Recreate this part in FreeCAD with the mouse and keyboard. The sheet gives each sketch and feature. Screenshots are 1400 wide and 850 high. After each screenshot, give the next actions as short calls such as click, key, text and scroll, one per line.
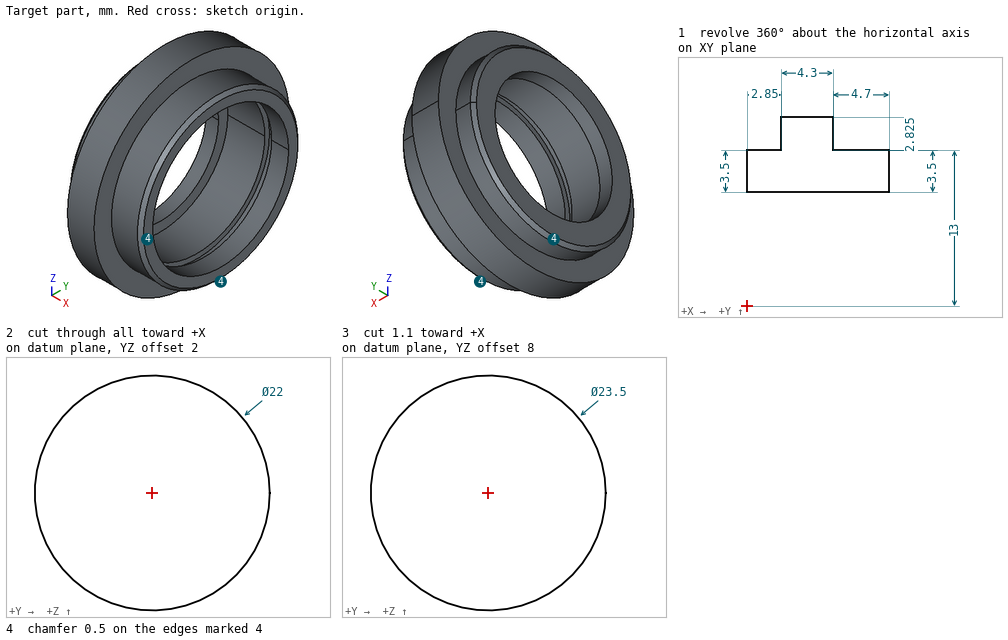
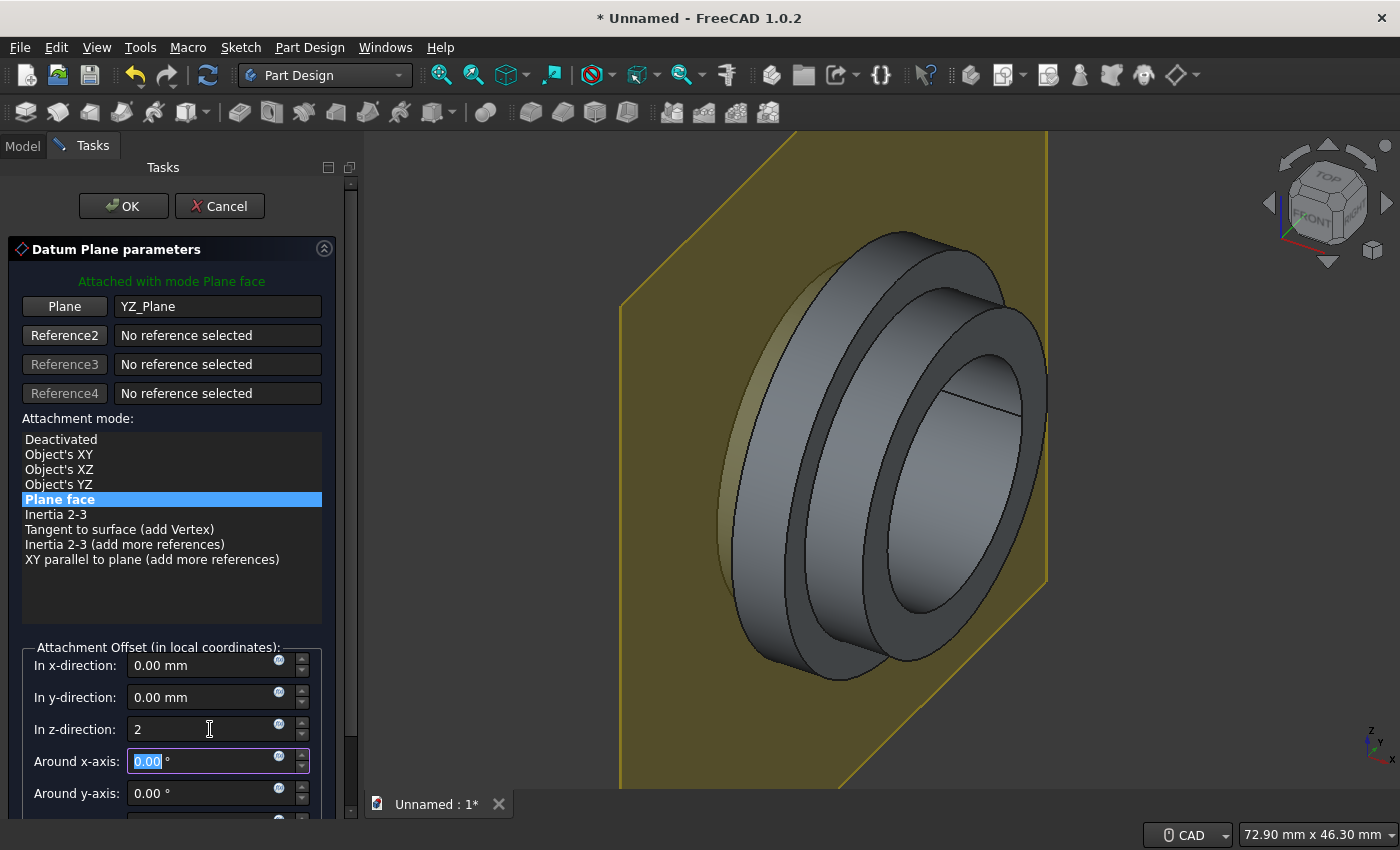
click(124, 206)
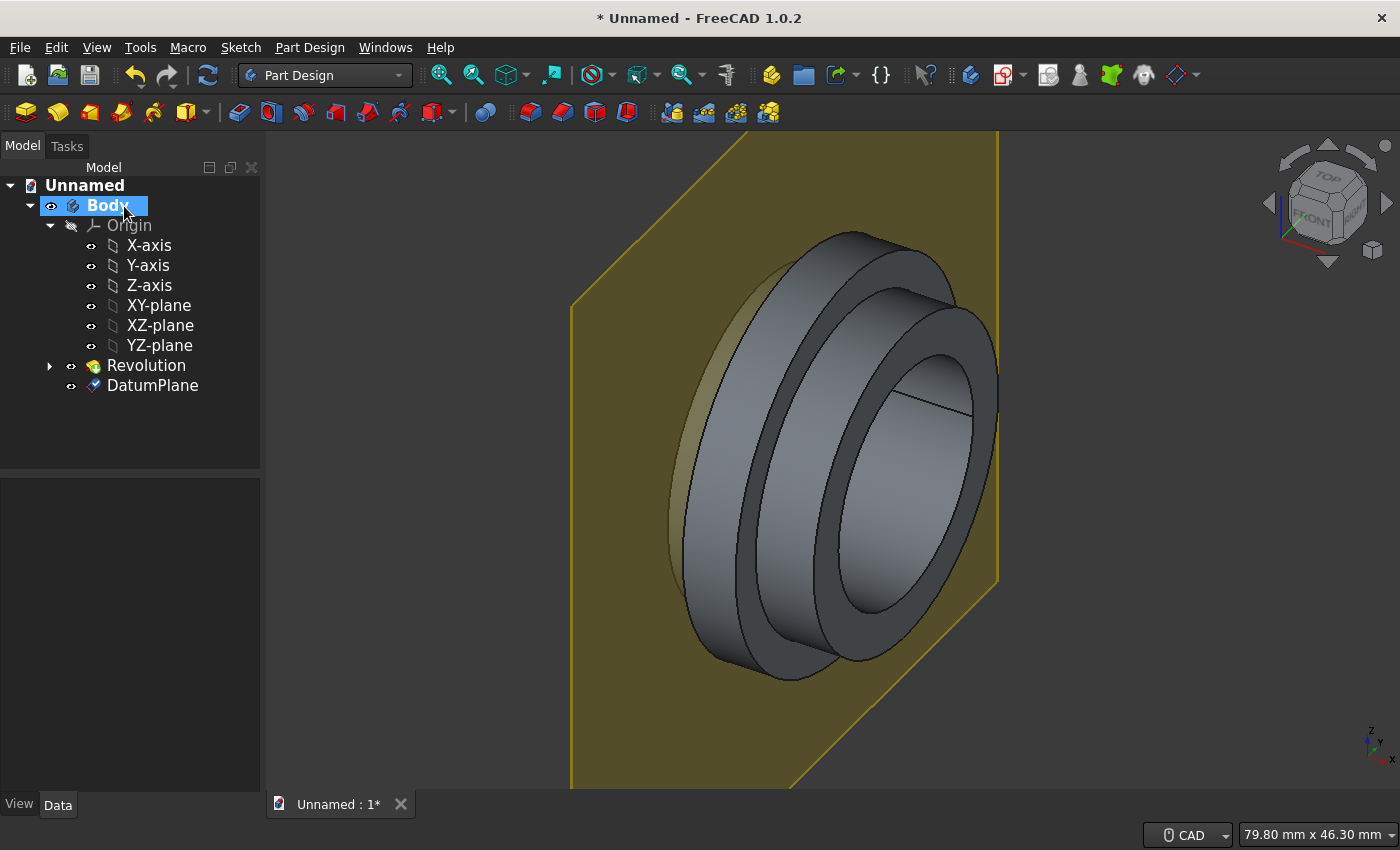
click(116, 386)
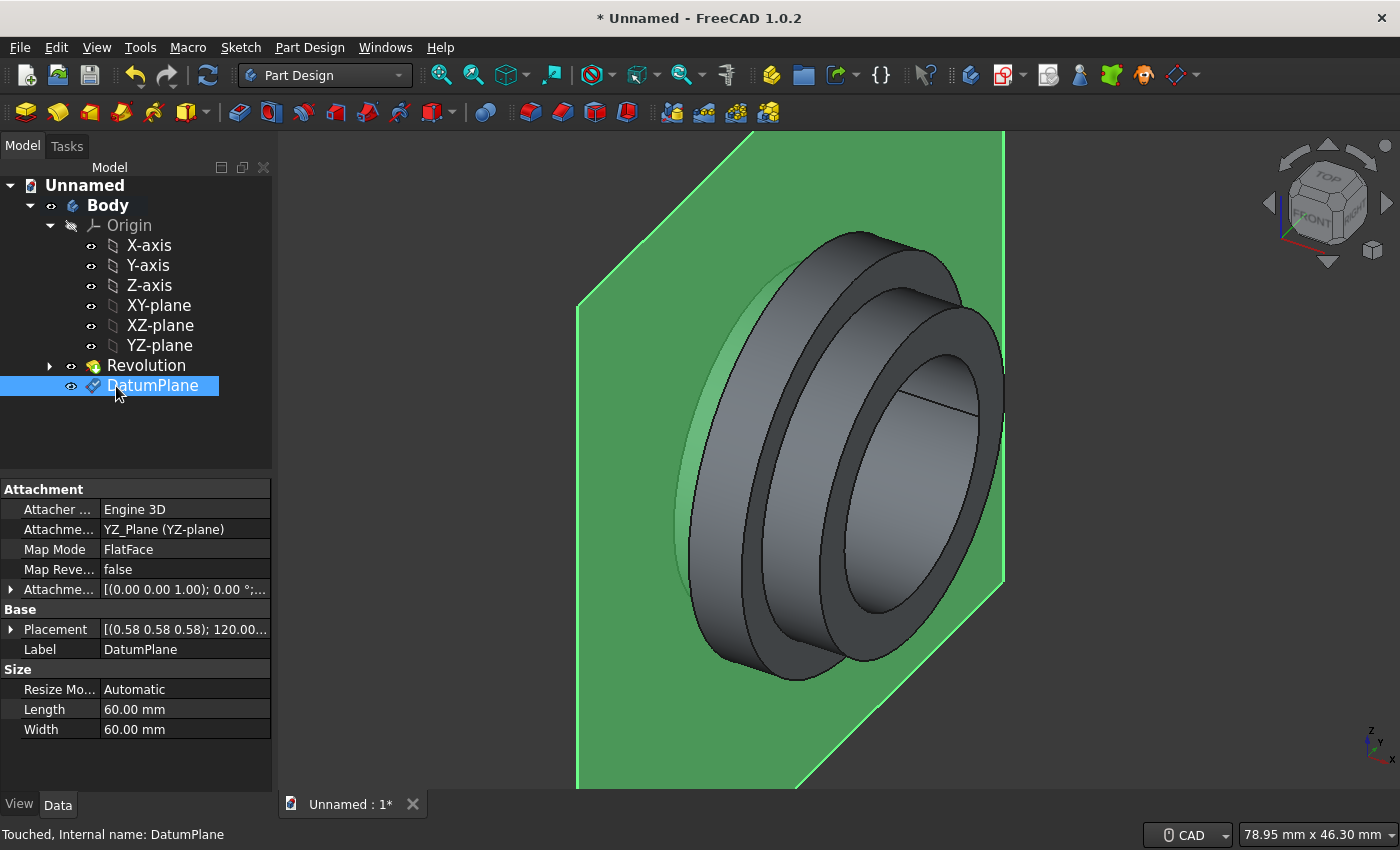
click(1004, 76)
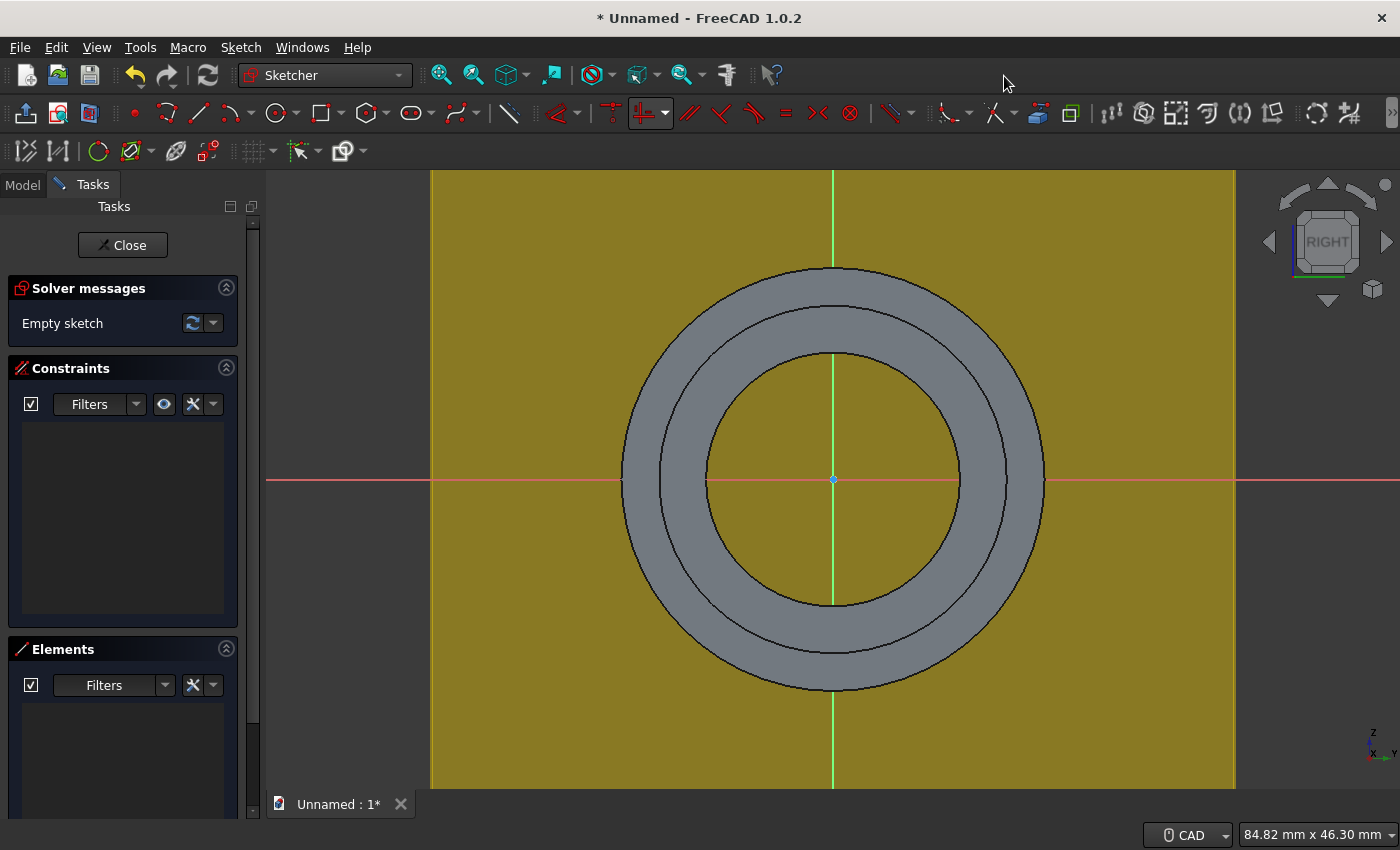
click(90, 114)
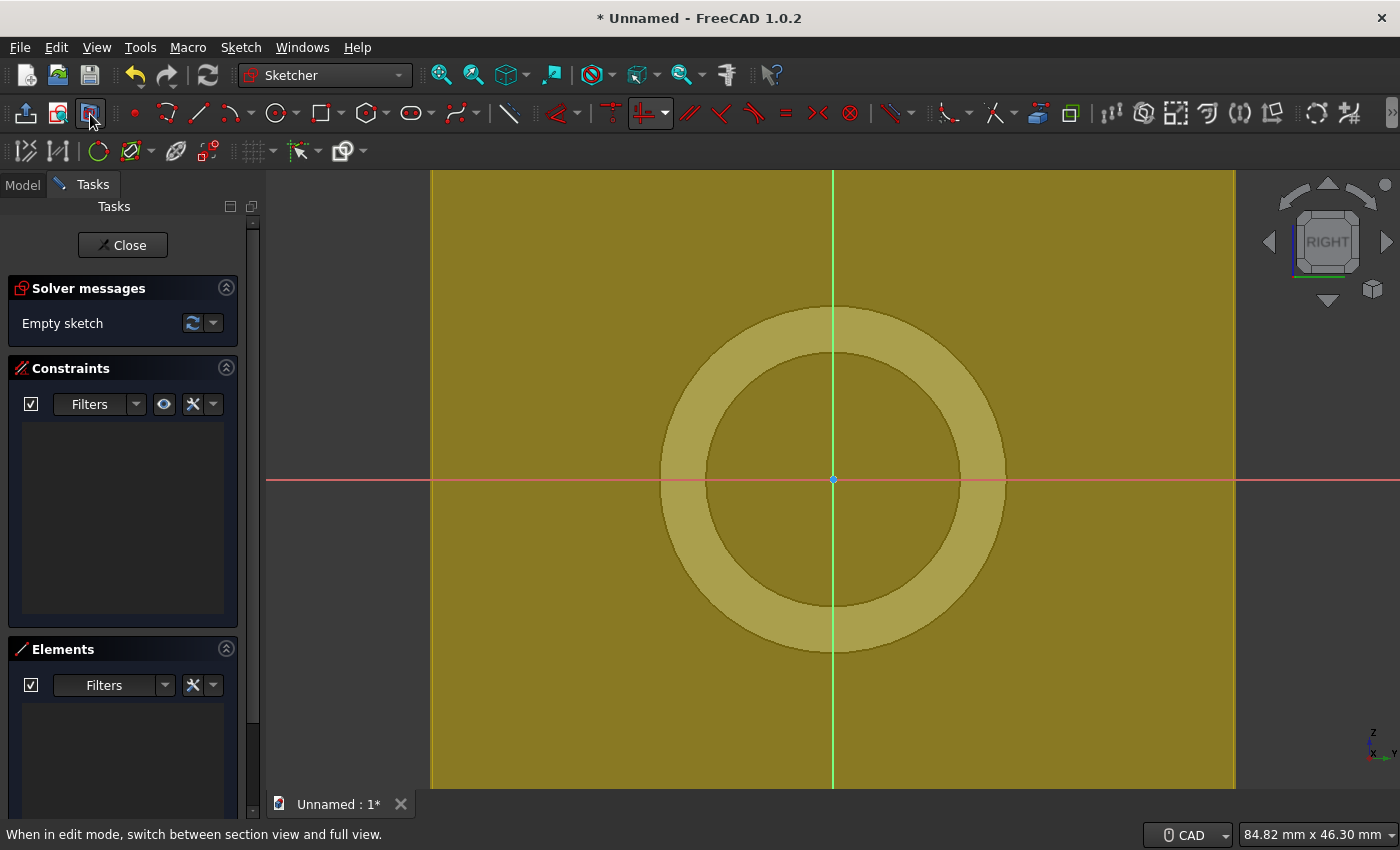
scroll(972, 480, up, 2)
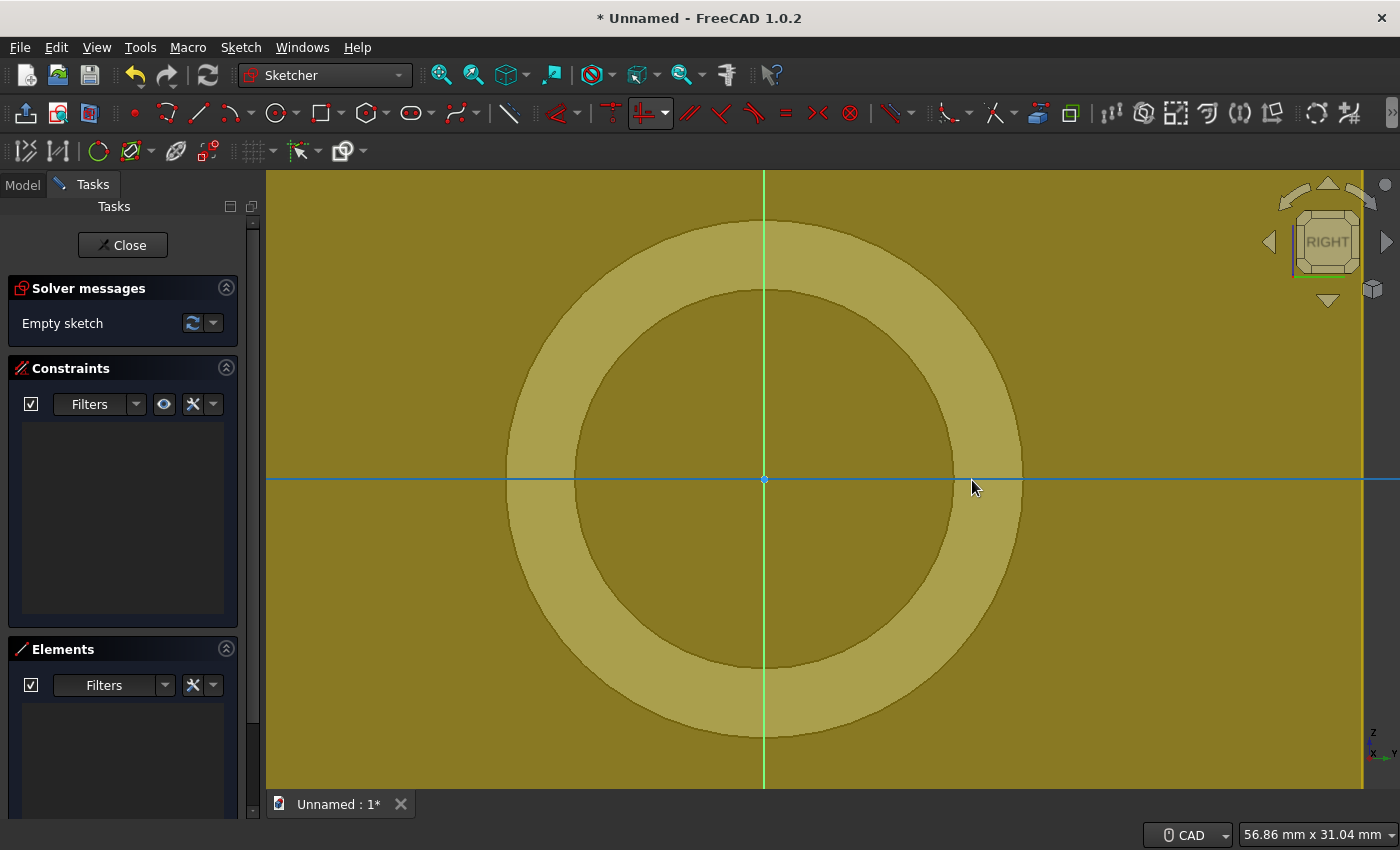
click(276, 114)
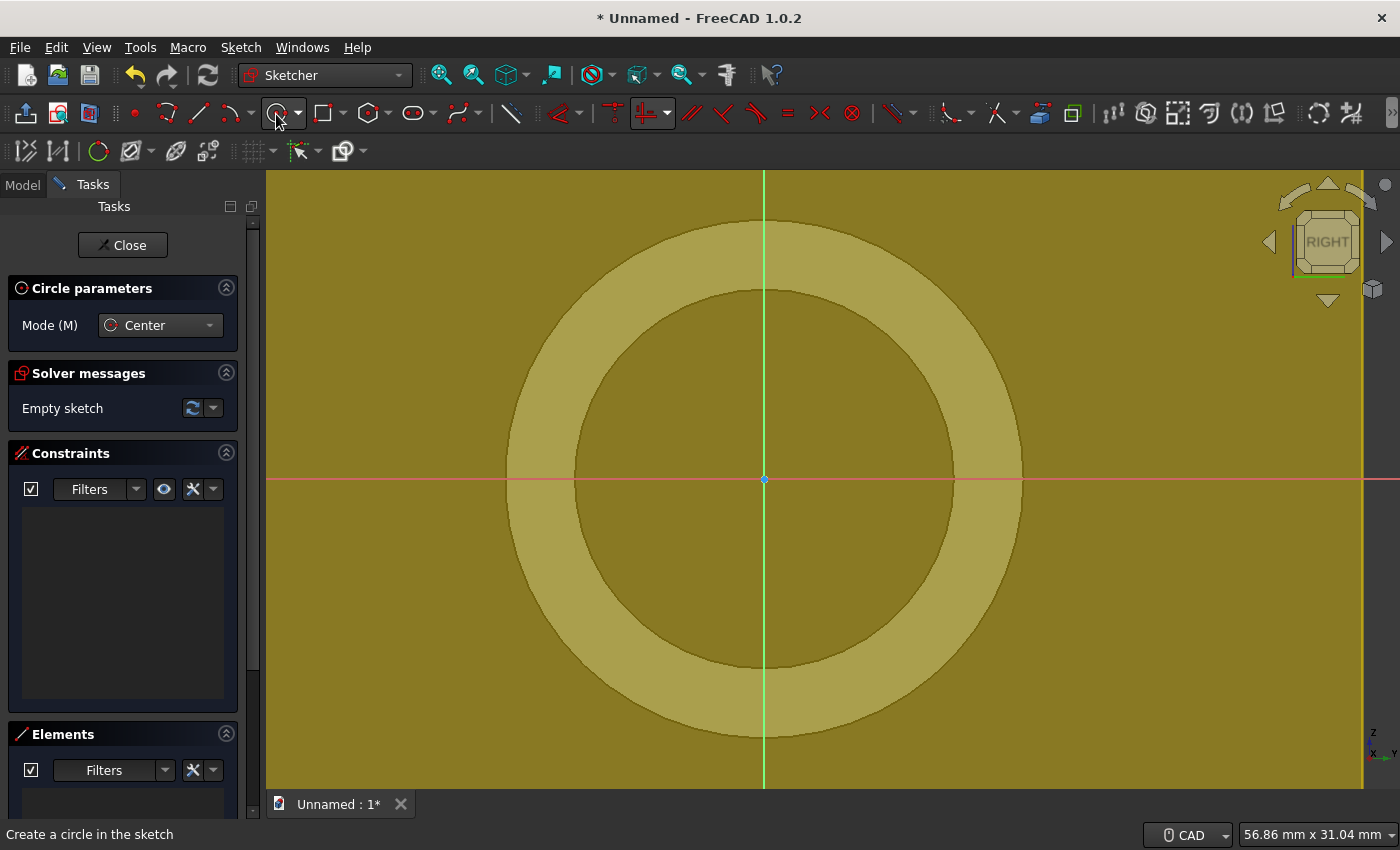
click(764, 479)
click(919, 324)
key(Escape)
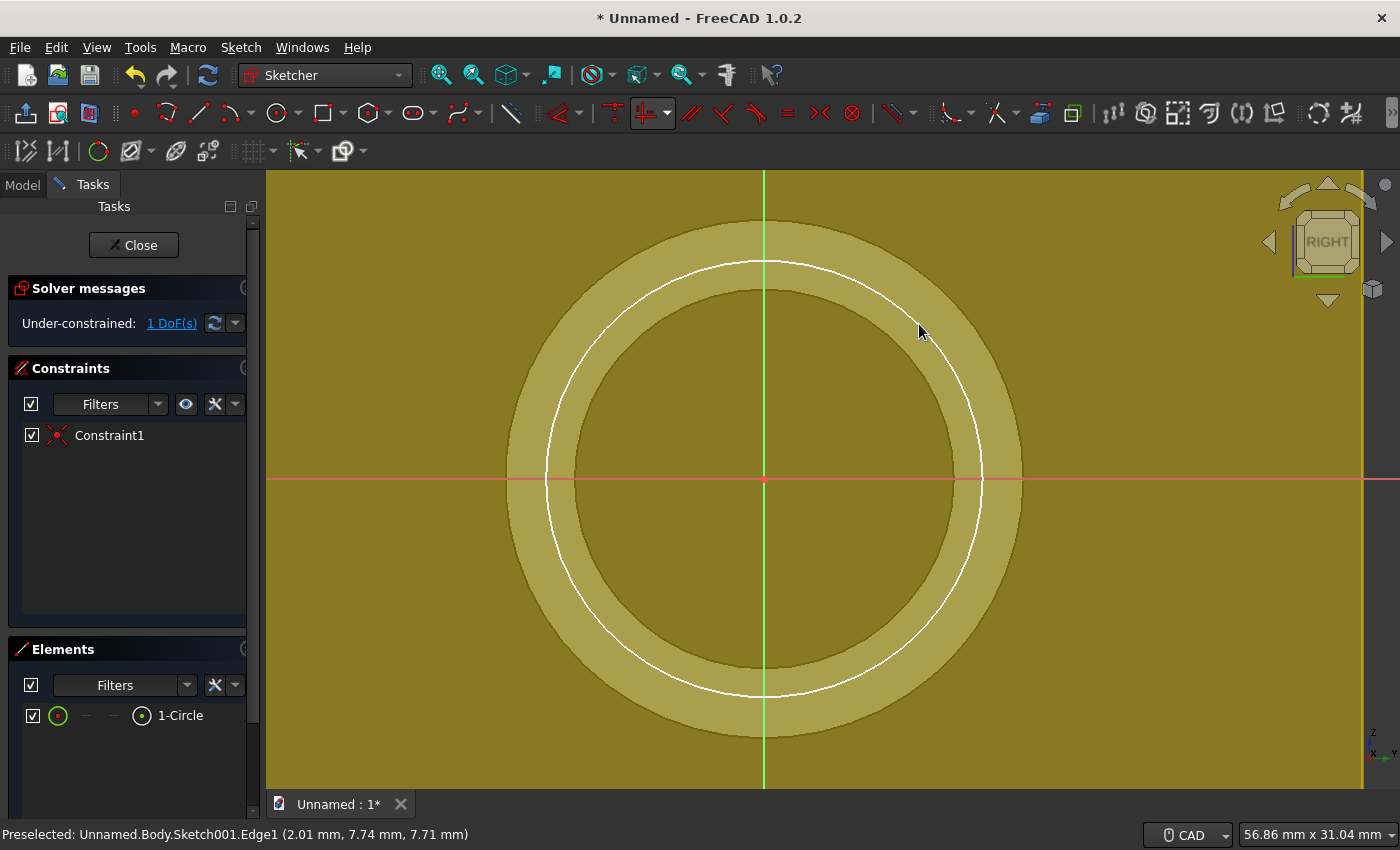
click(558, 114)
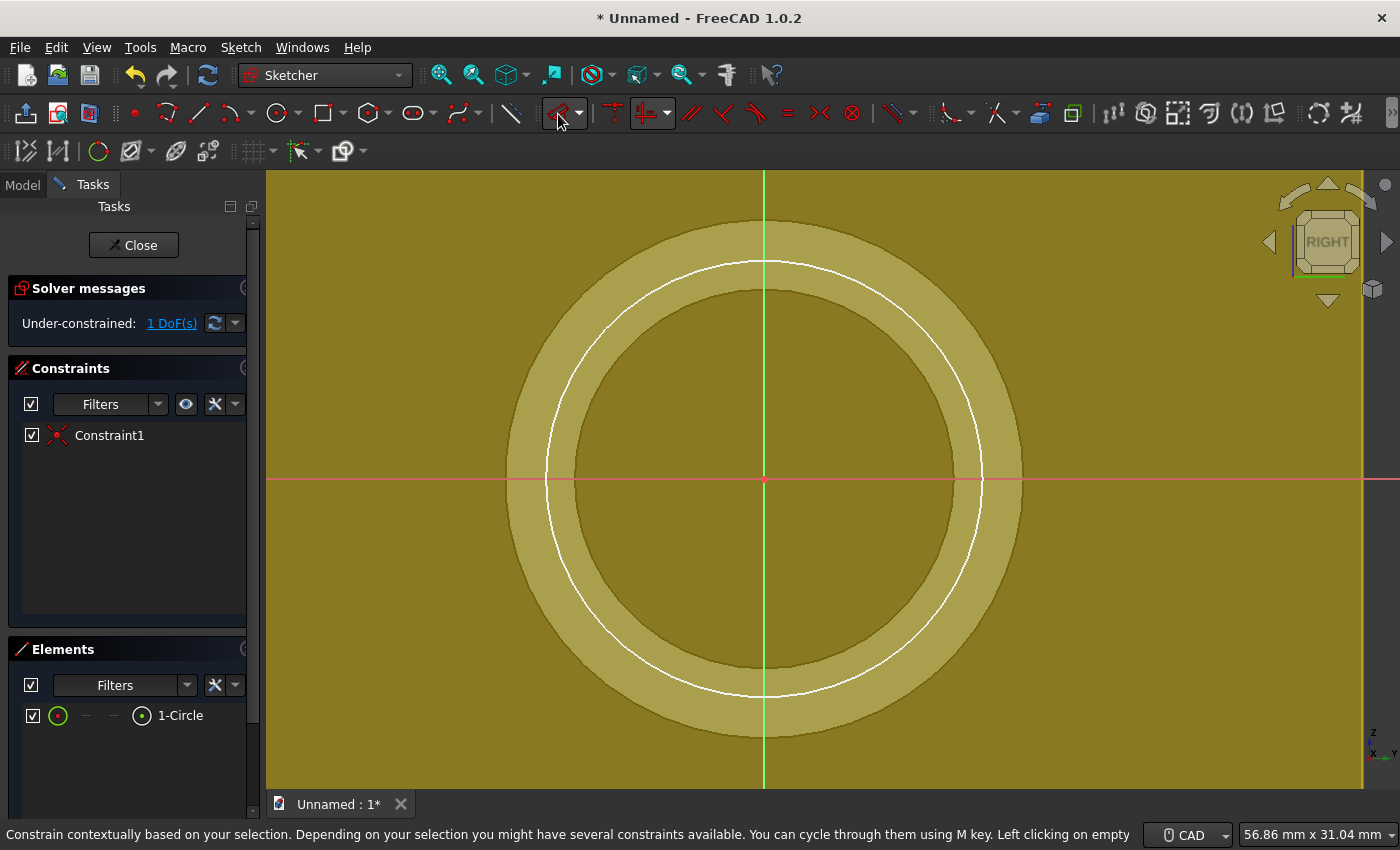
click(918, 324)
click(941, 301)